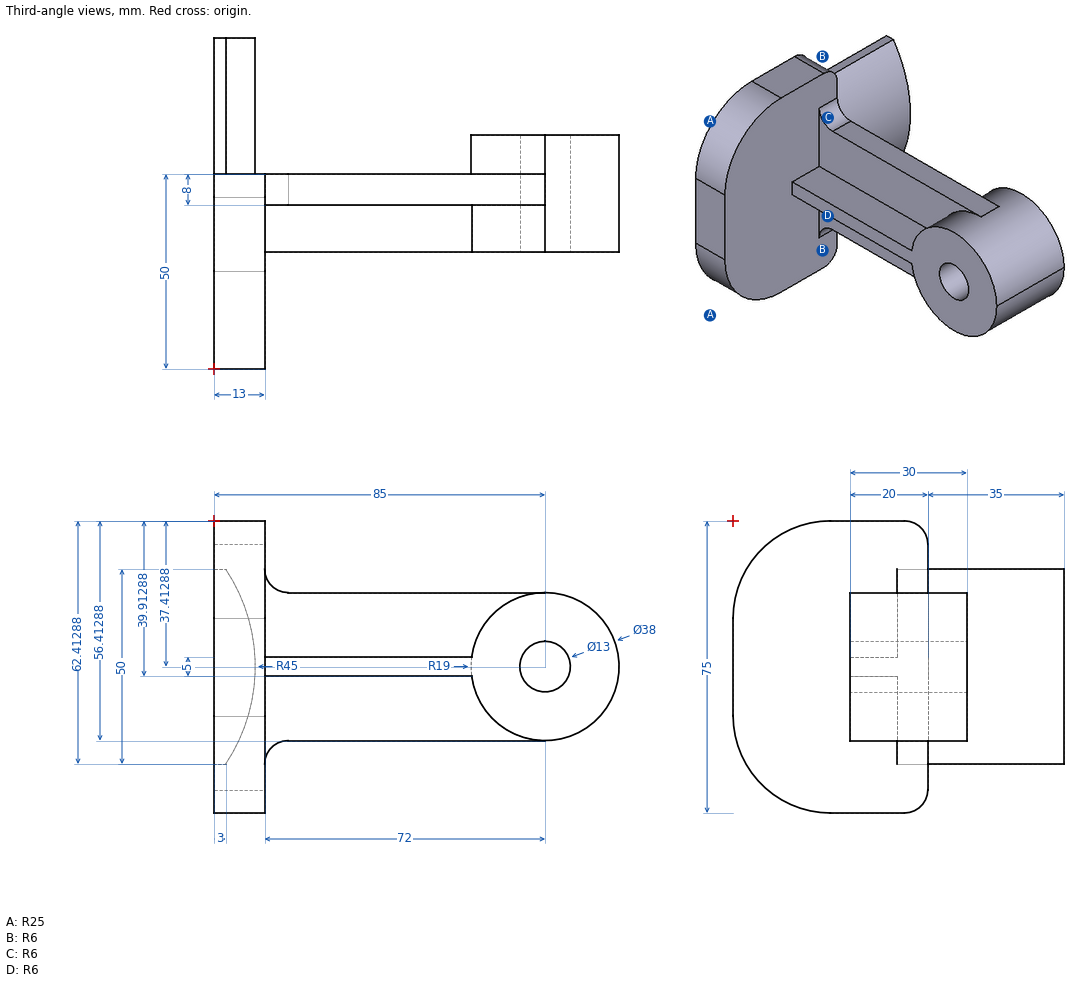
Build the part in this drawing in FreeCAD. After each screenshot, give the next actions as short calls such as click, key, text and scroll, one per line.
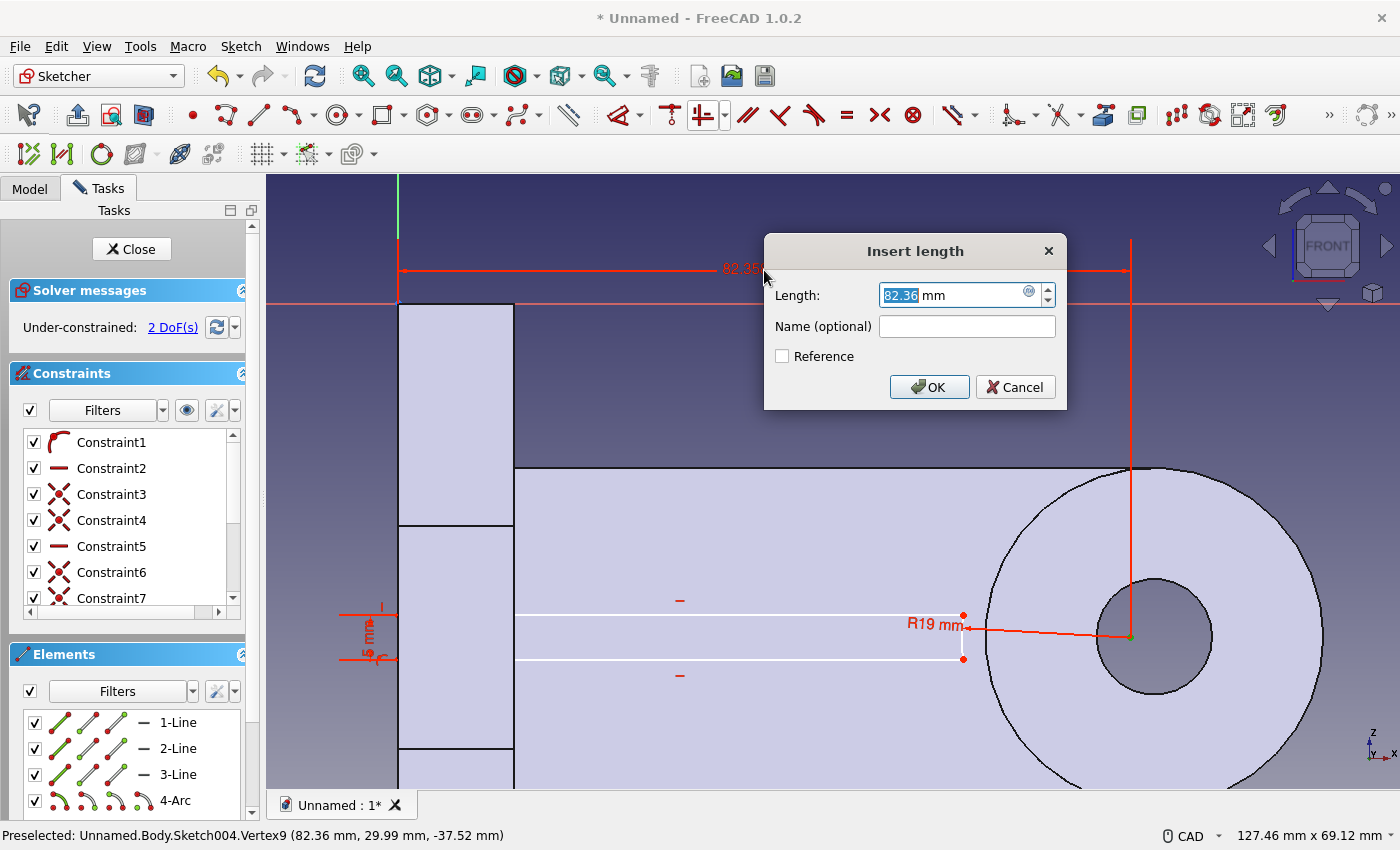
text(85)
key(Return)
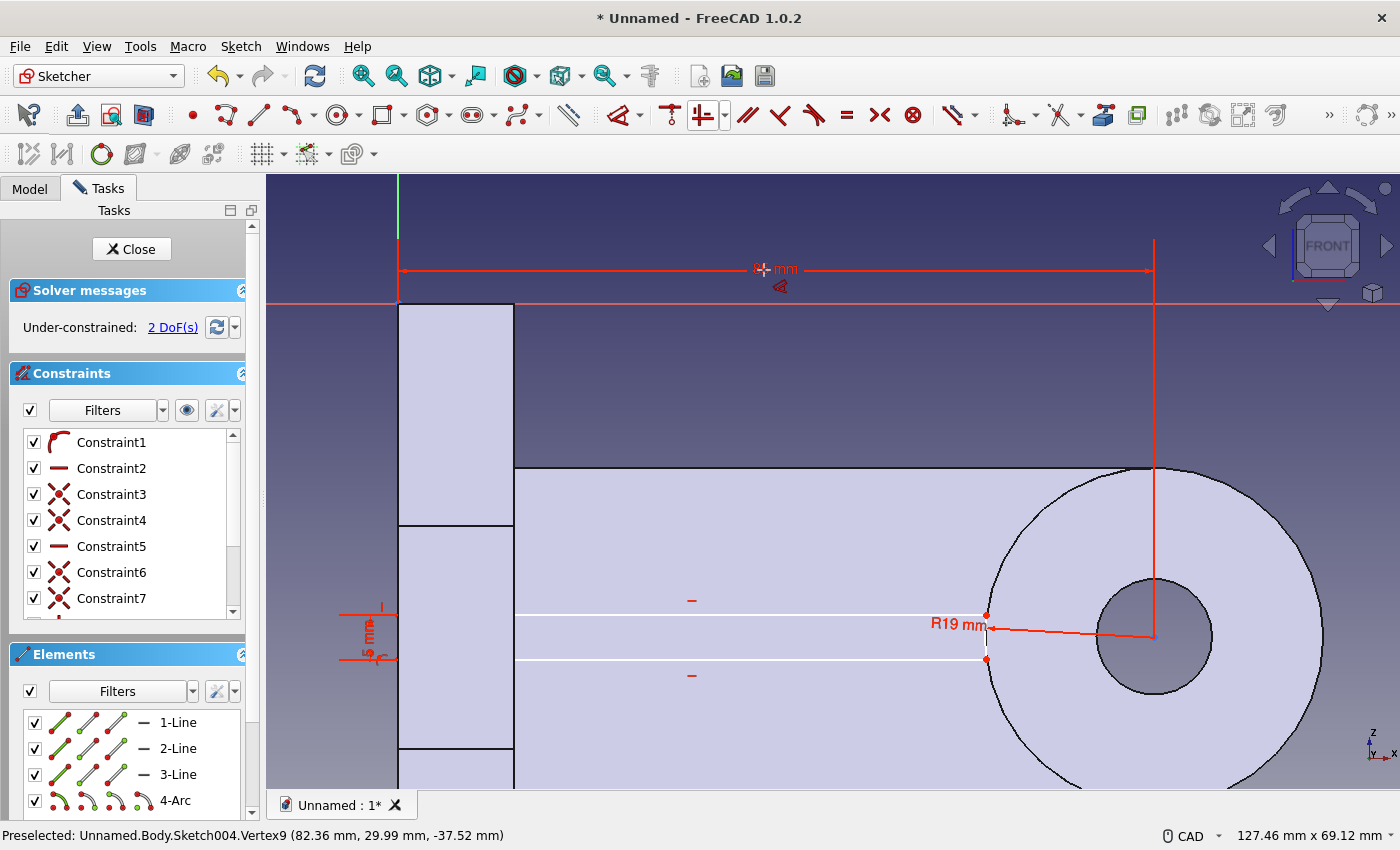
click(987, 660)
click(364, 482)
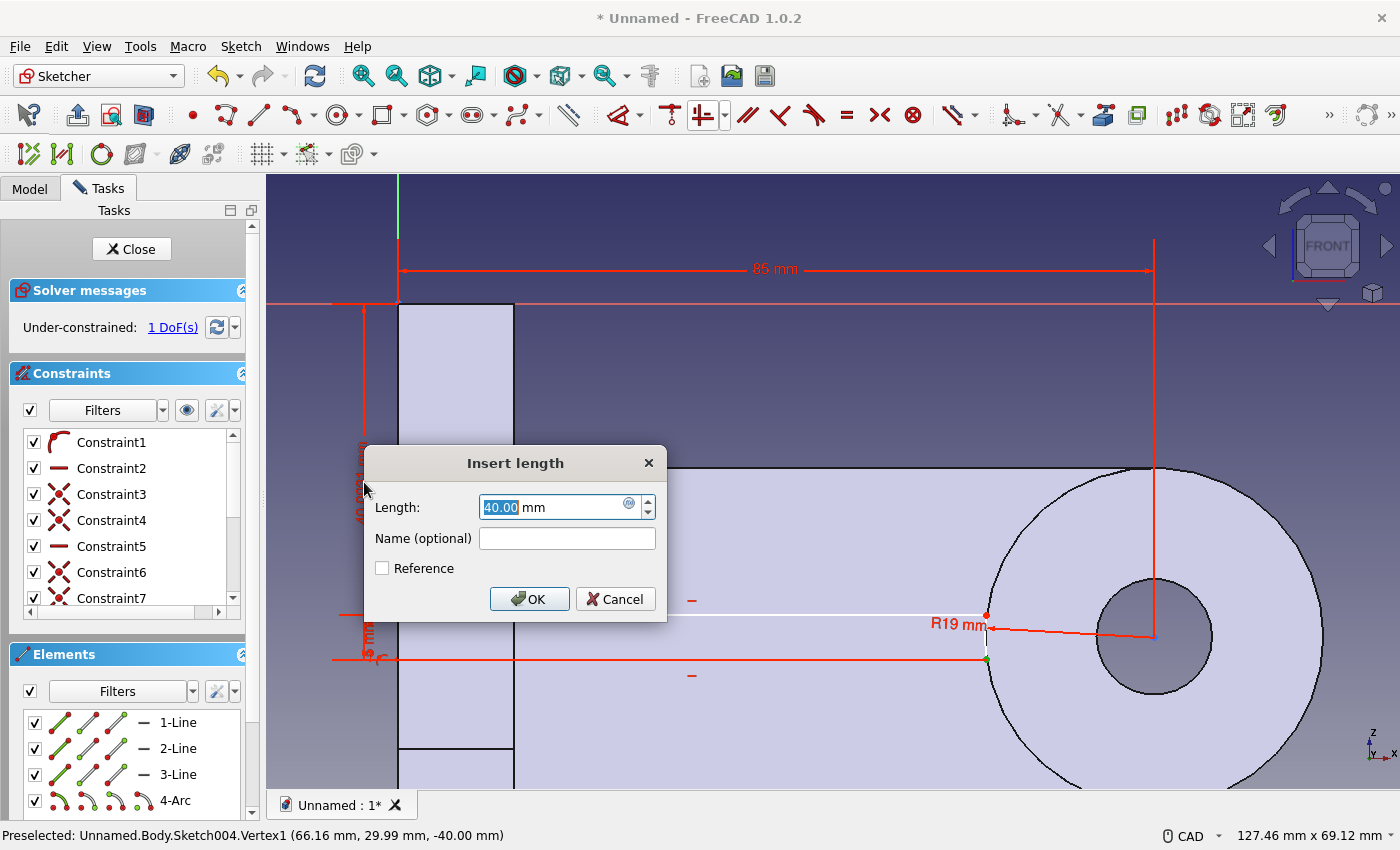
text(39.91288)
key(Return)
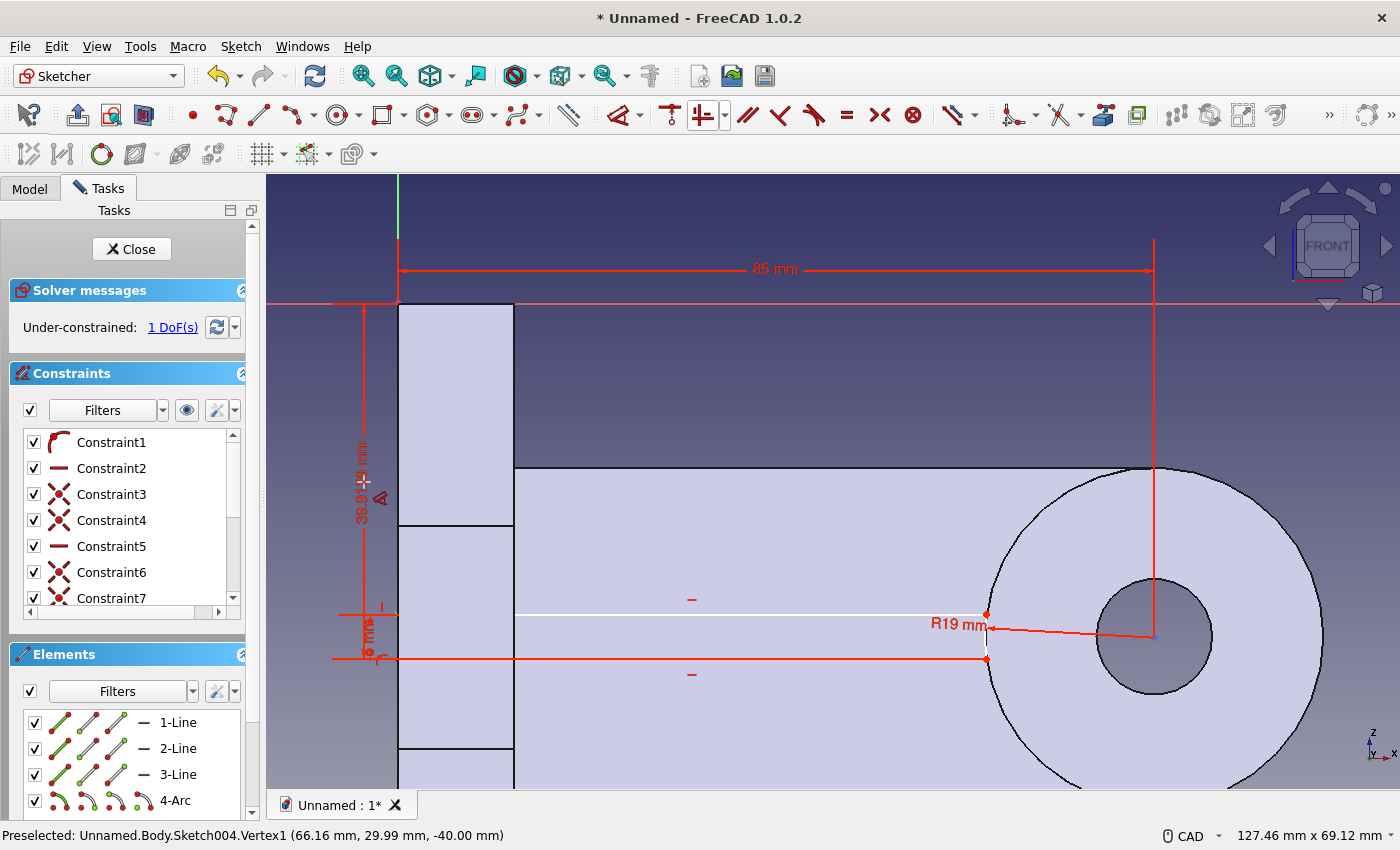
click(1154, 638)
click(1188, 471)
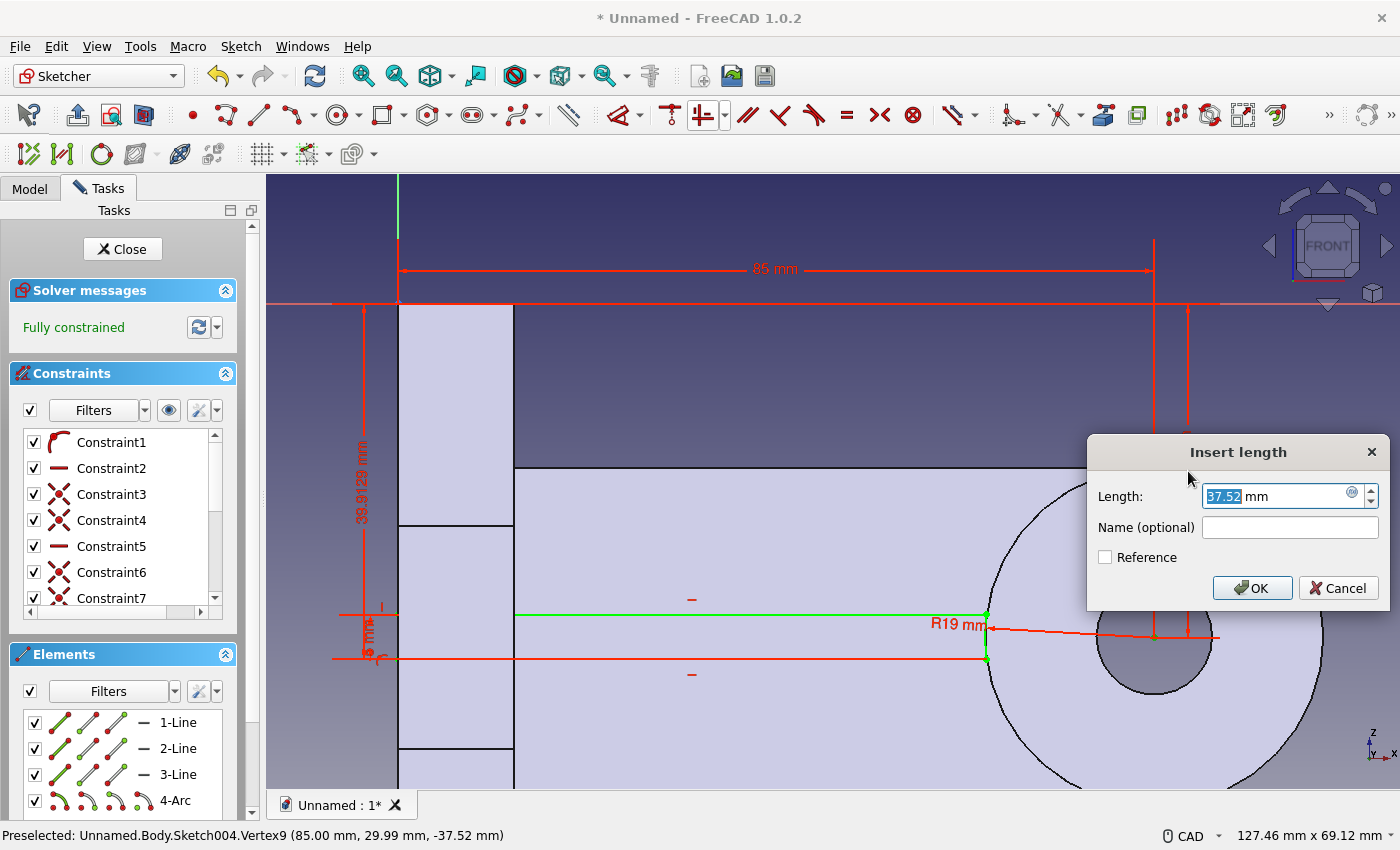
text(37.41288)
key(Return)
key(Escape)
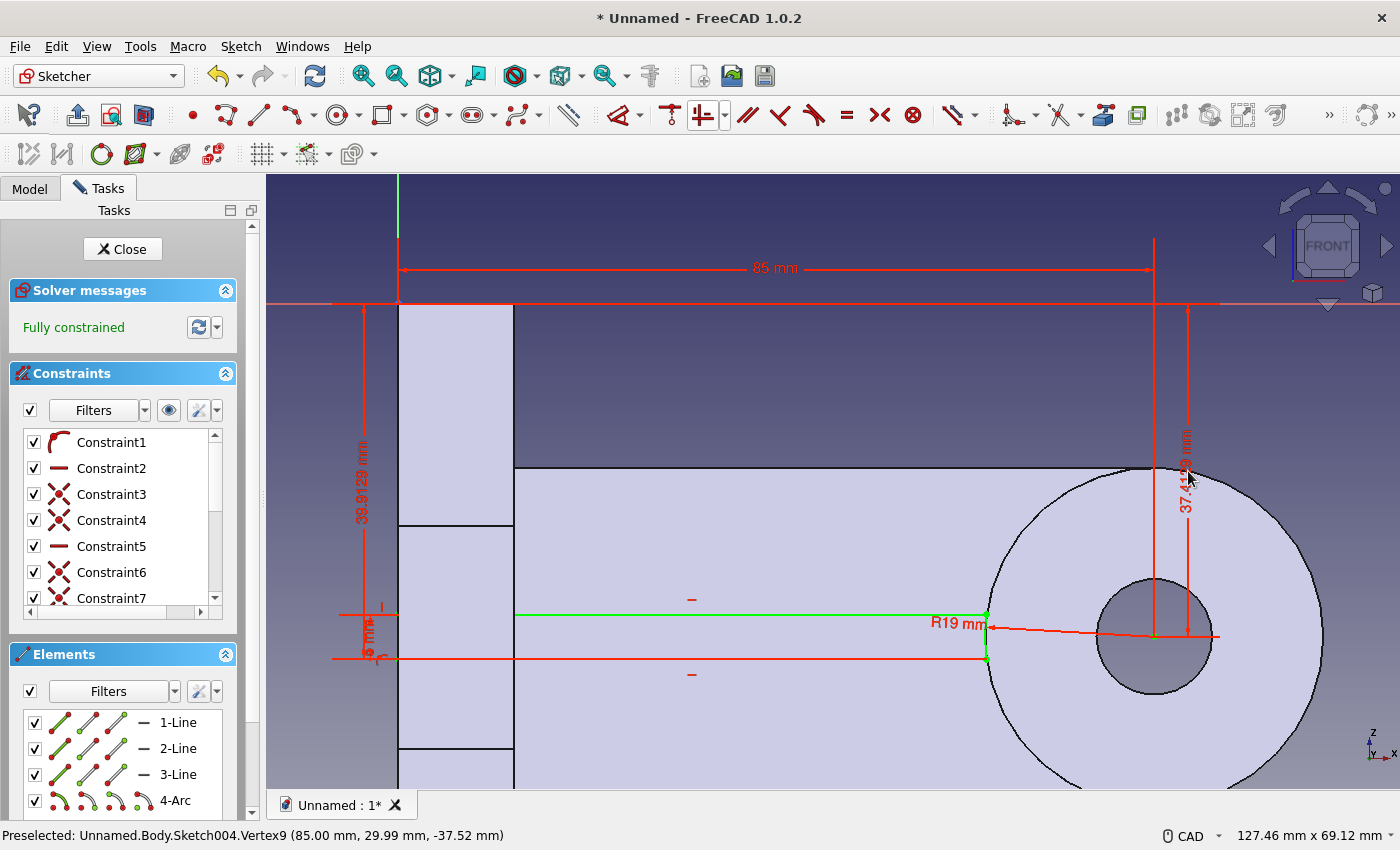
click(123, 249)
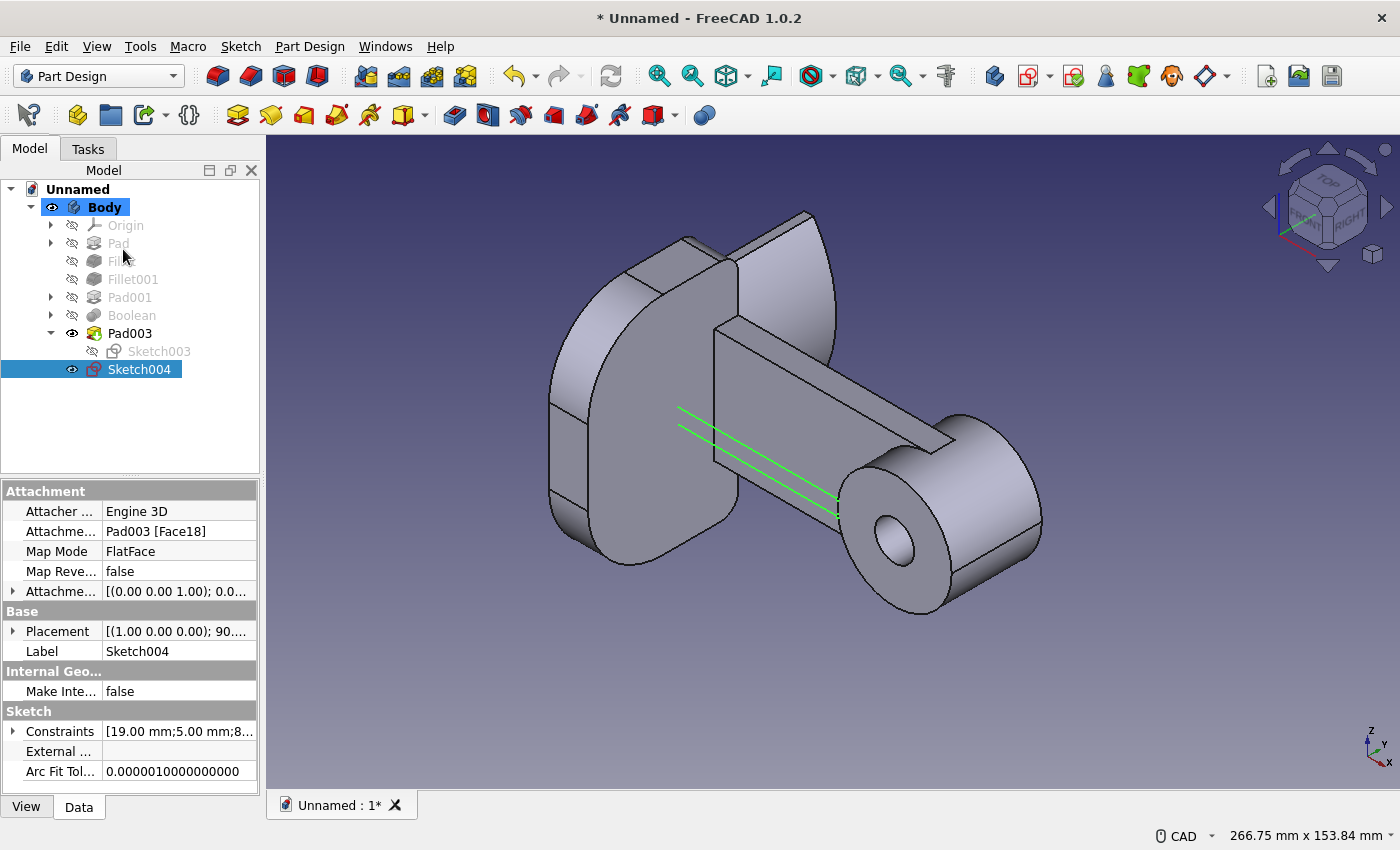
click(238, 116)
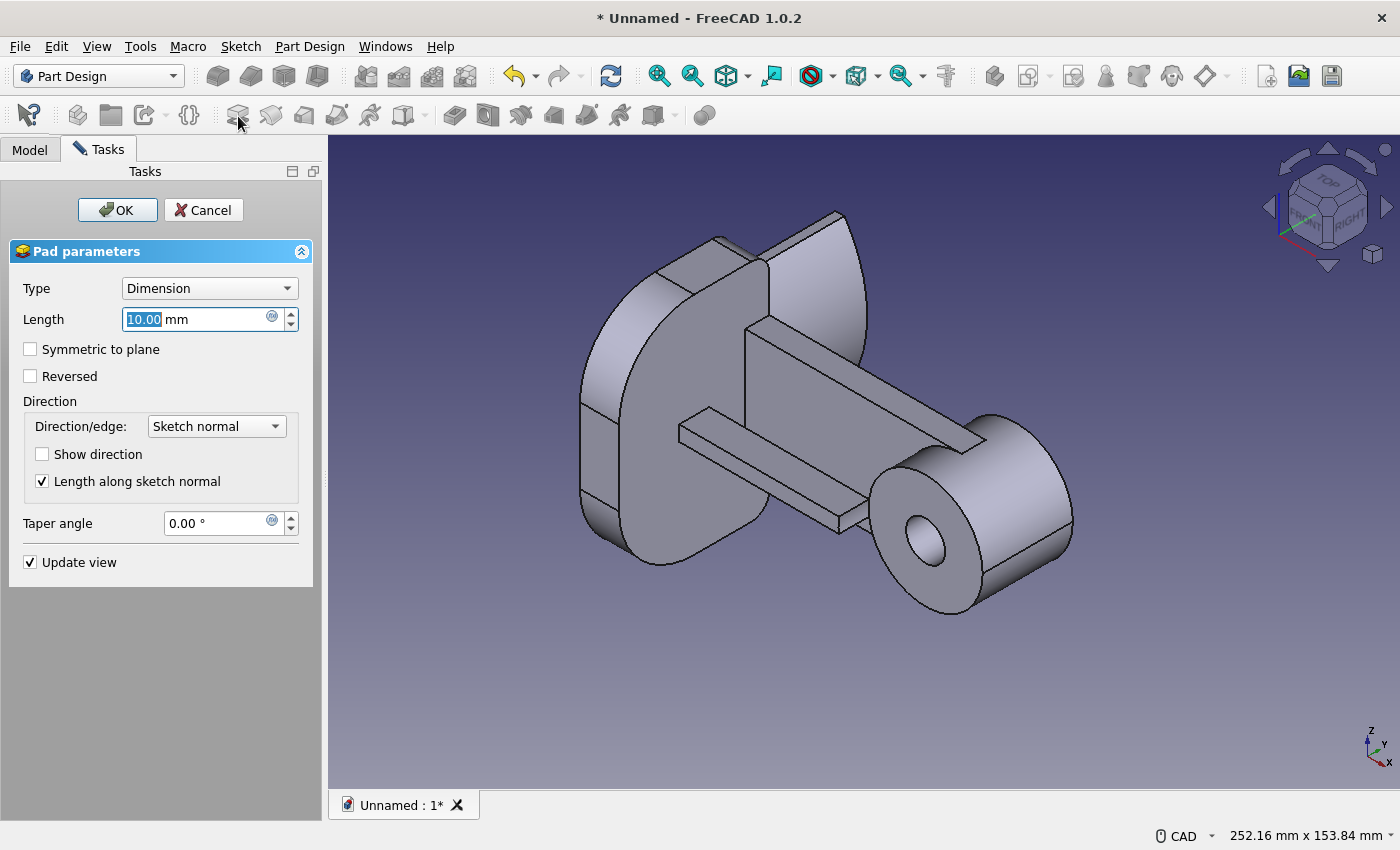
text(20)
key(Tab)